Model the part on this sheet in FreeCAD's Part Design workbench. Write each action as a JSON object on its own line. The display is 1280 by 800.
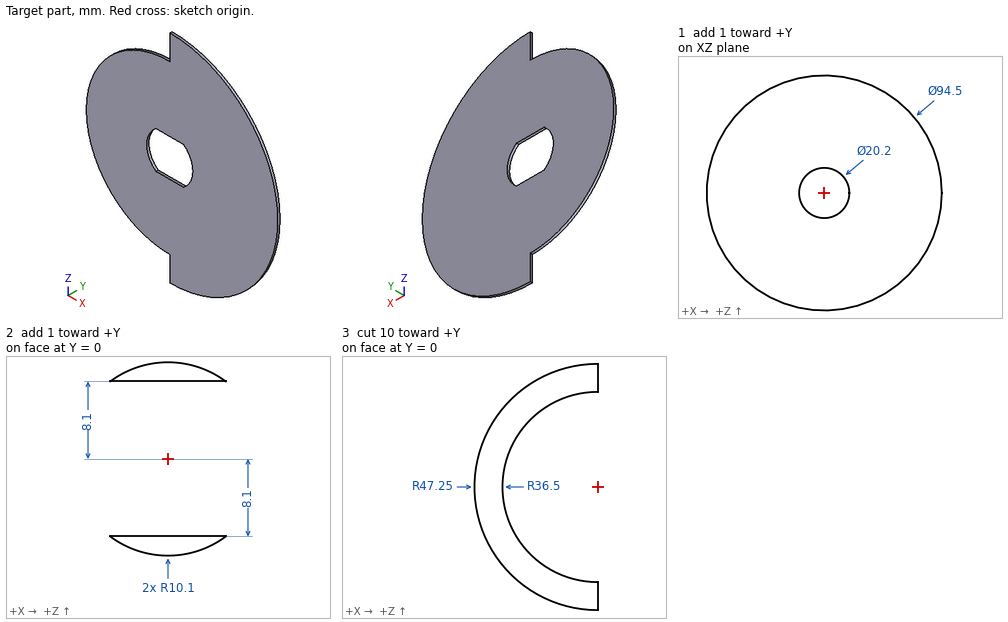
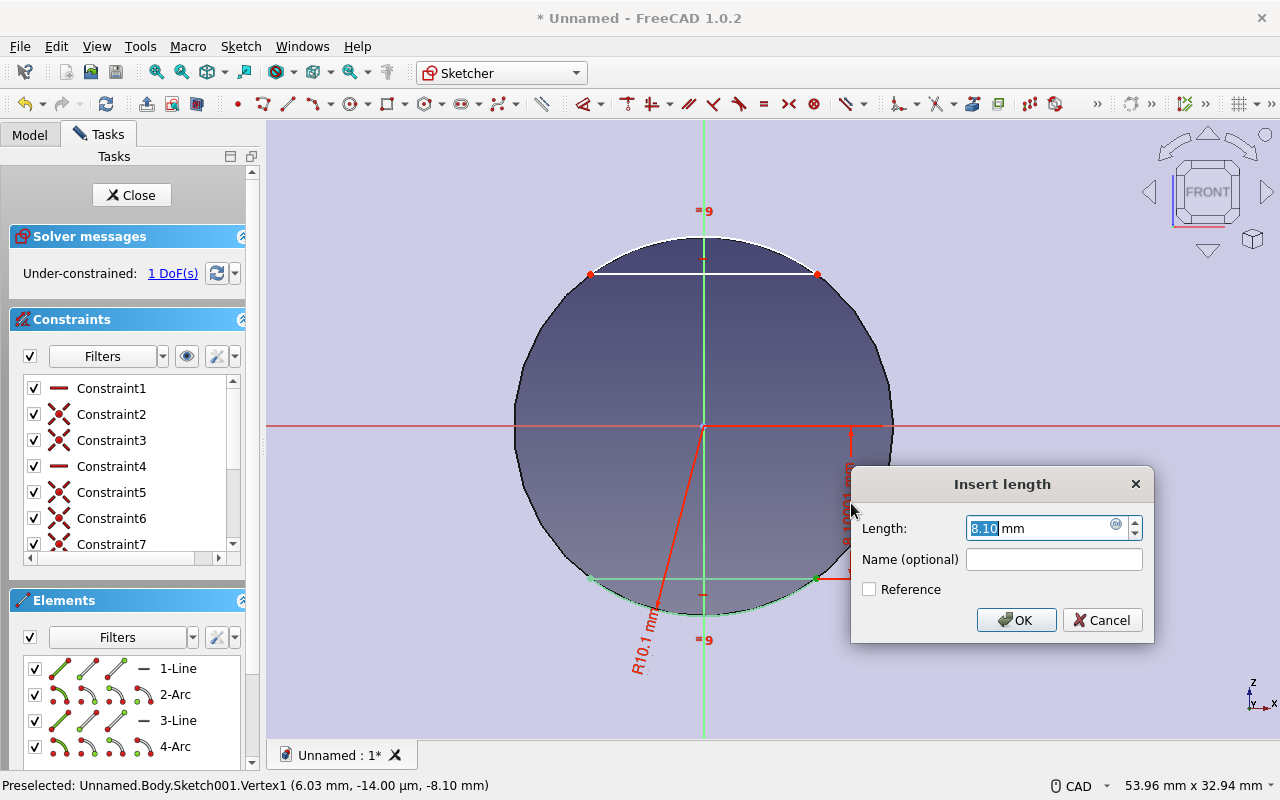
{"action": "type", "text": "8.1"}
{"action": "key", "text": "Return"}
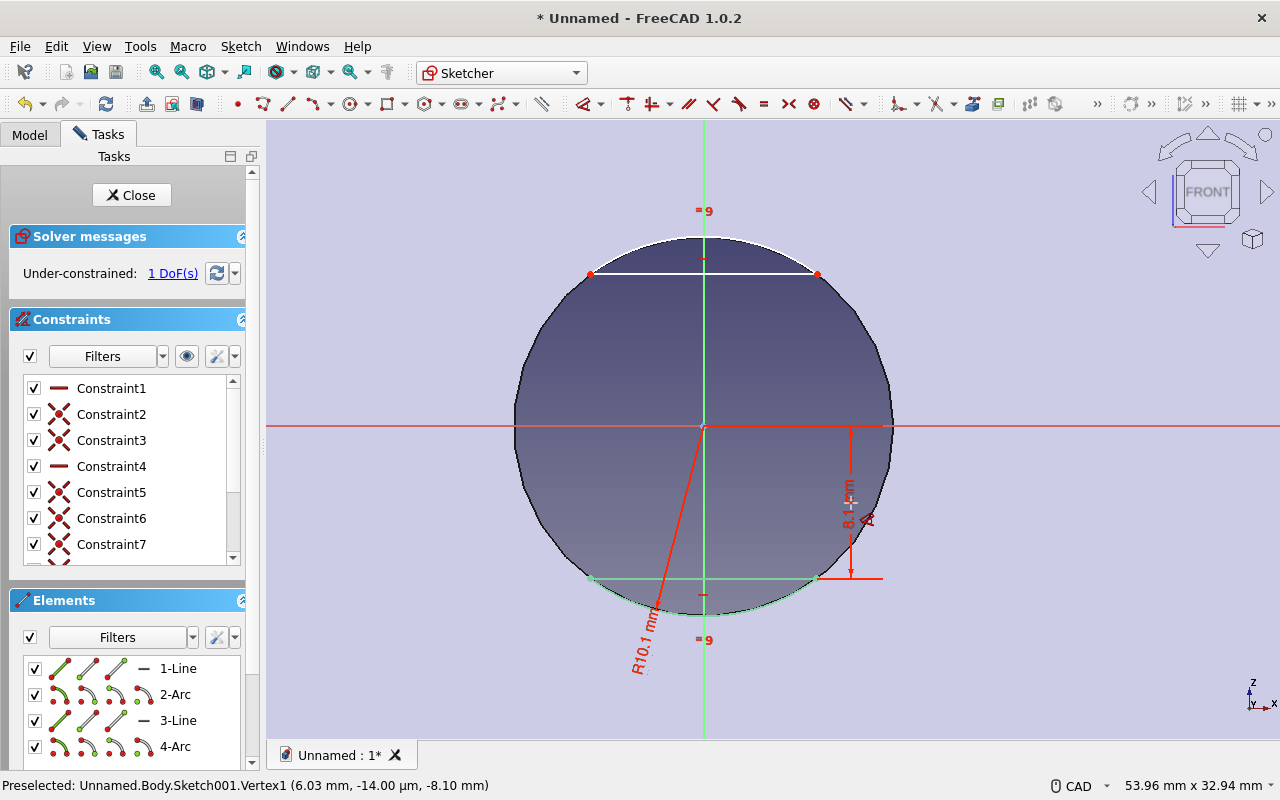
{"action": "left_click", "coordinate": [590, 274]}
{"action": "left_click", "coordinate": [556, 350]}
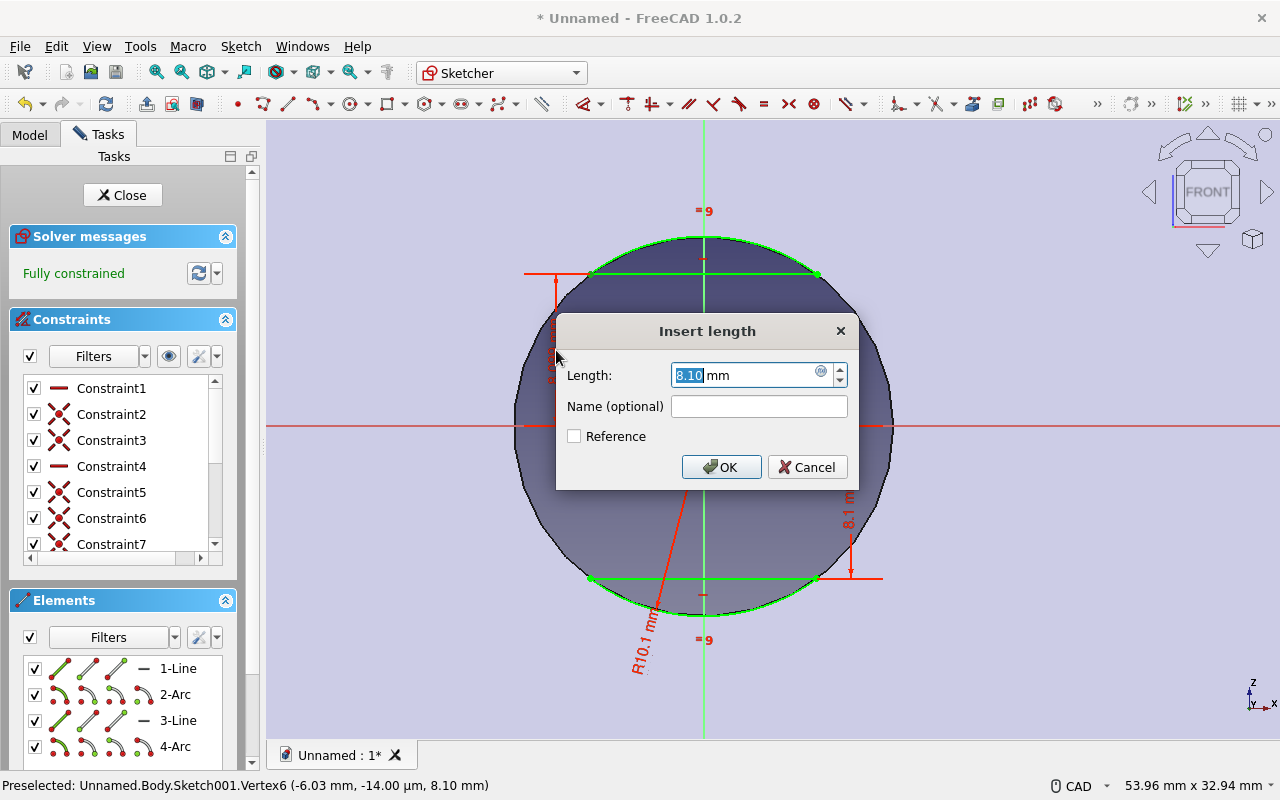
{"action": "type", "text": "8.1"}
{"action": "key", "text": "Return"}
{"action": "key", "text": "Escape"}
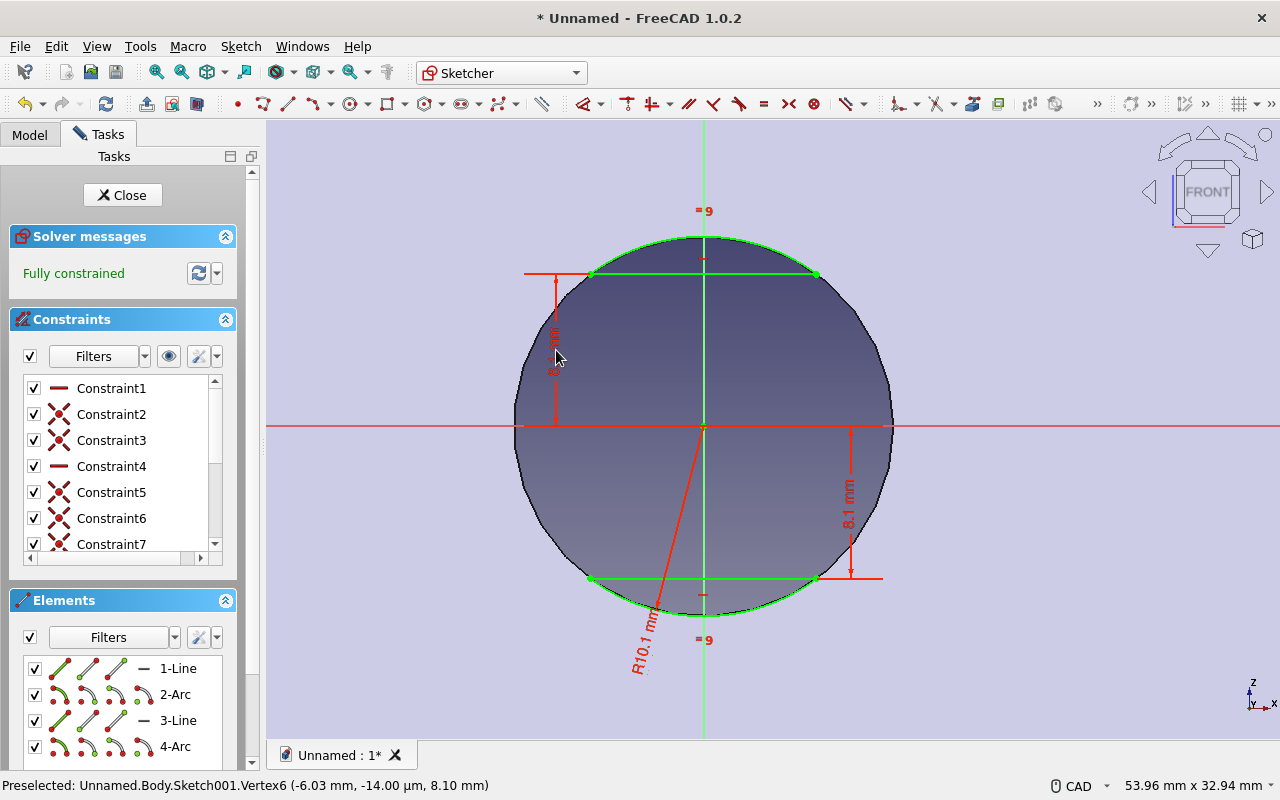
{"action": "left_click", "coordinate": [123, 195]}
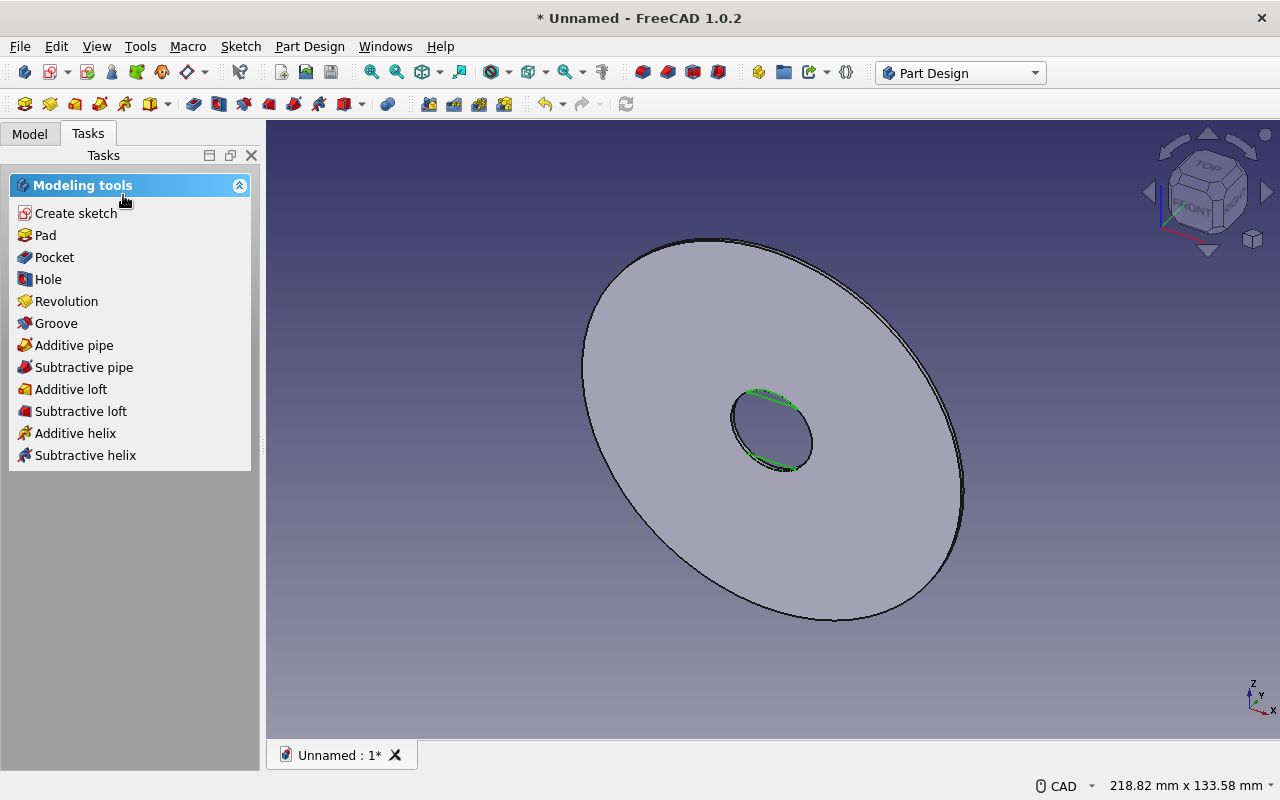
{"action": "left_click", "coordinate": [25, 104]}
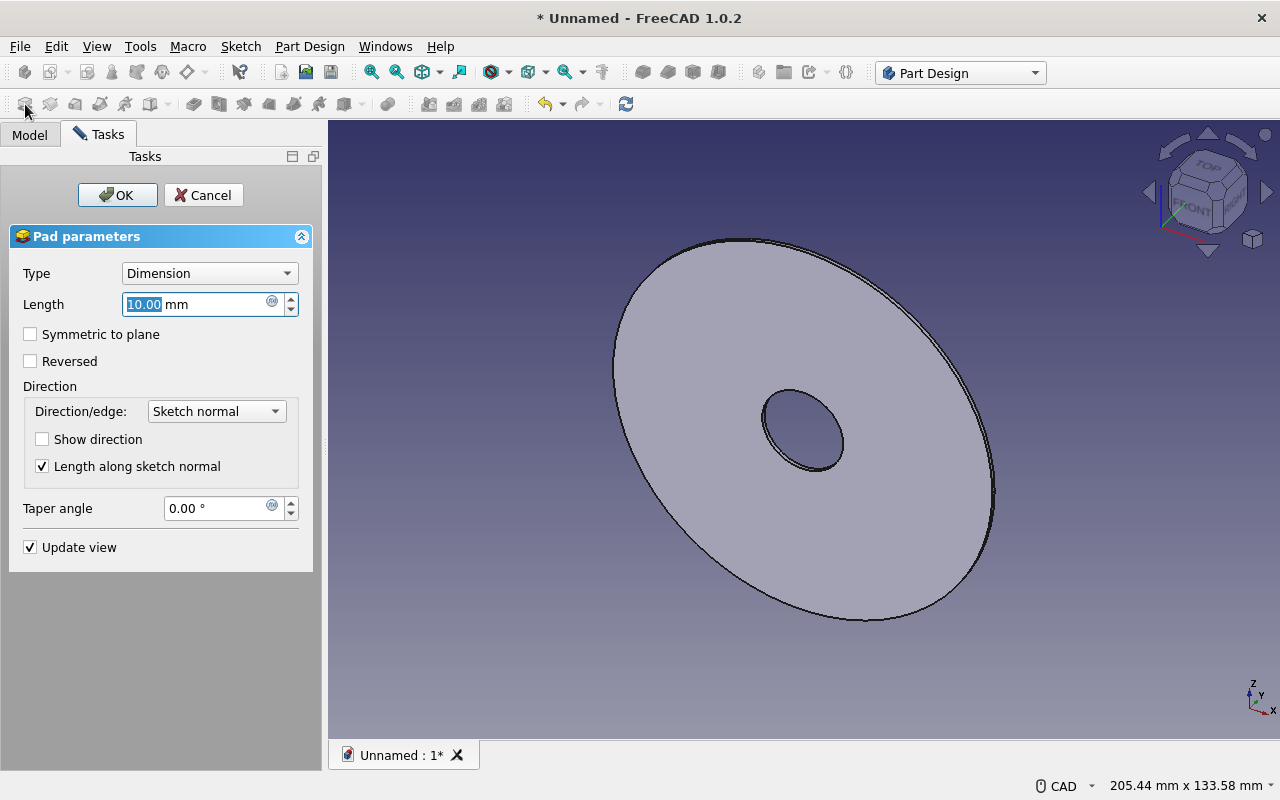
{"action": "type", "text": "1"}
{"action": "key", "text": "Tab"}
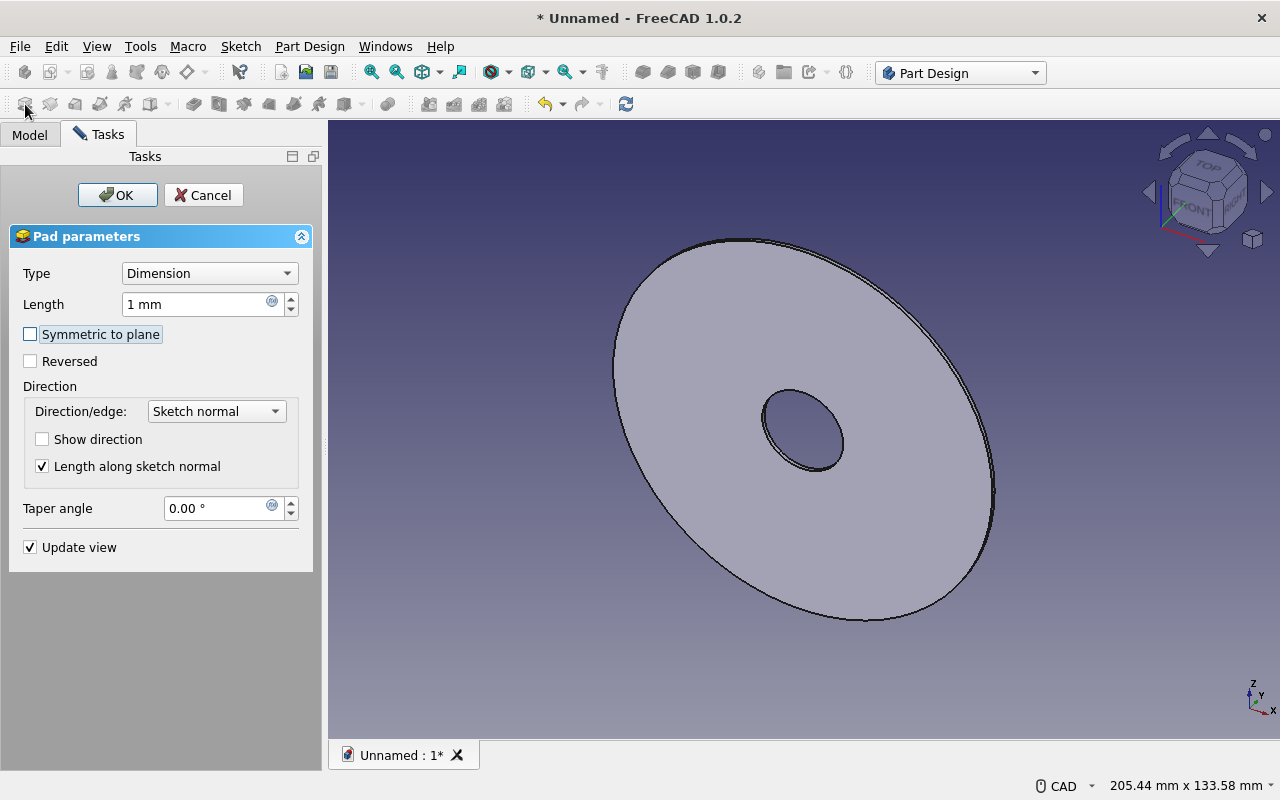
{"action": "left_click", "coordinate": [31, 361]}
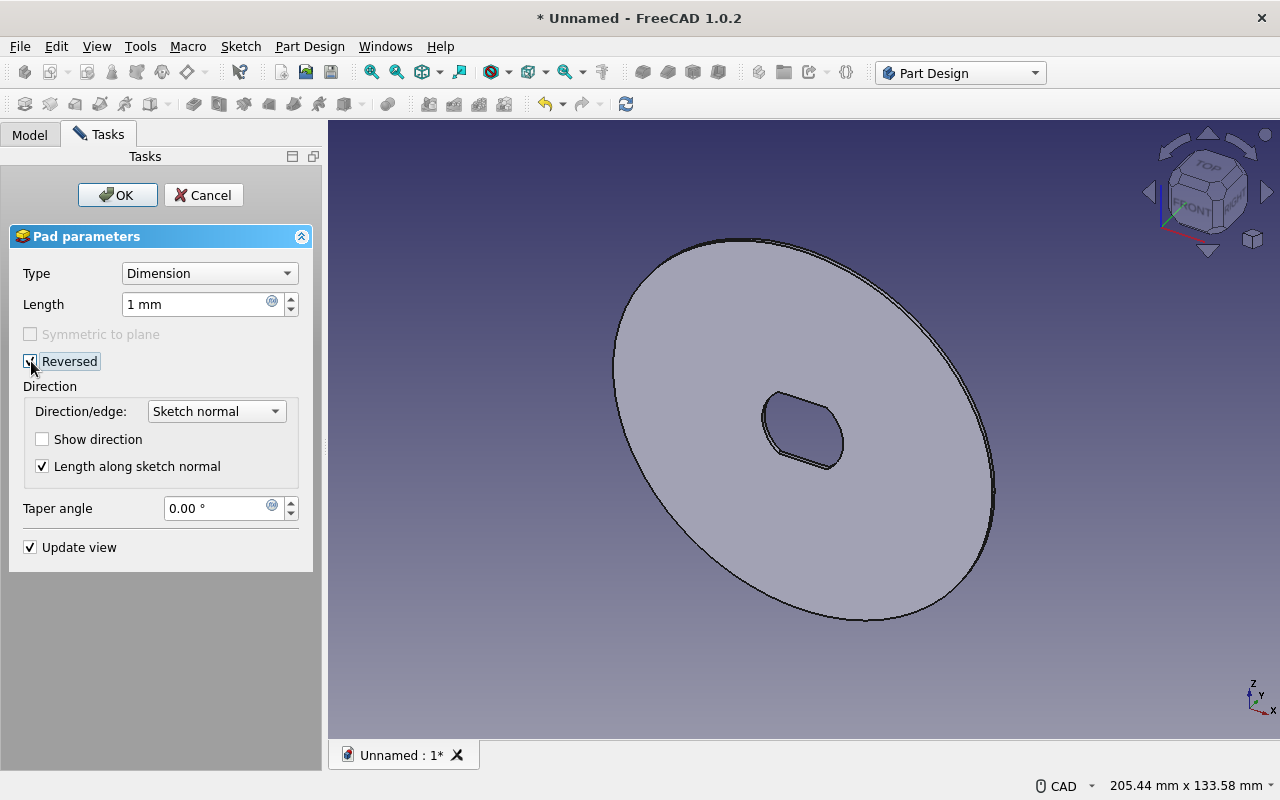
{"action": "left_click", "coordinate": [118, 195]}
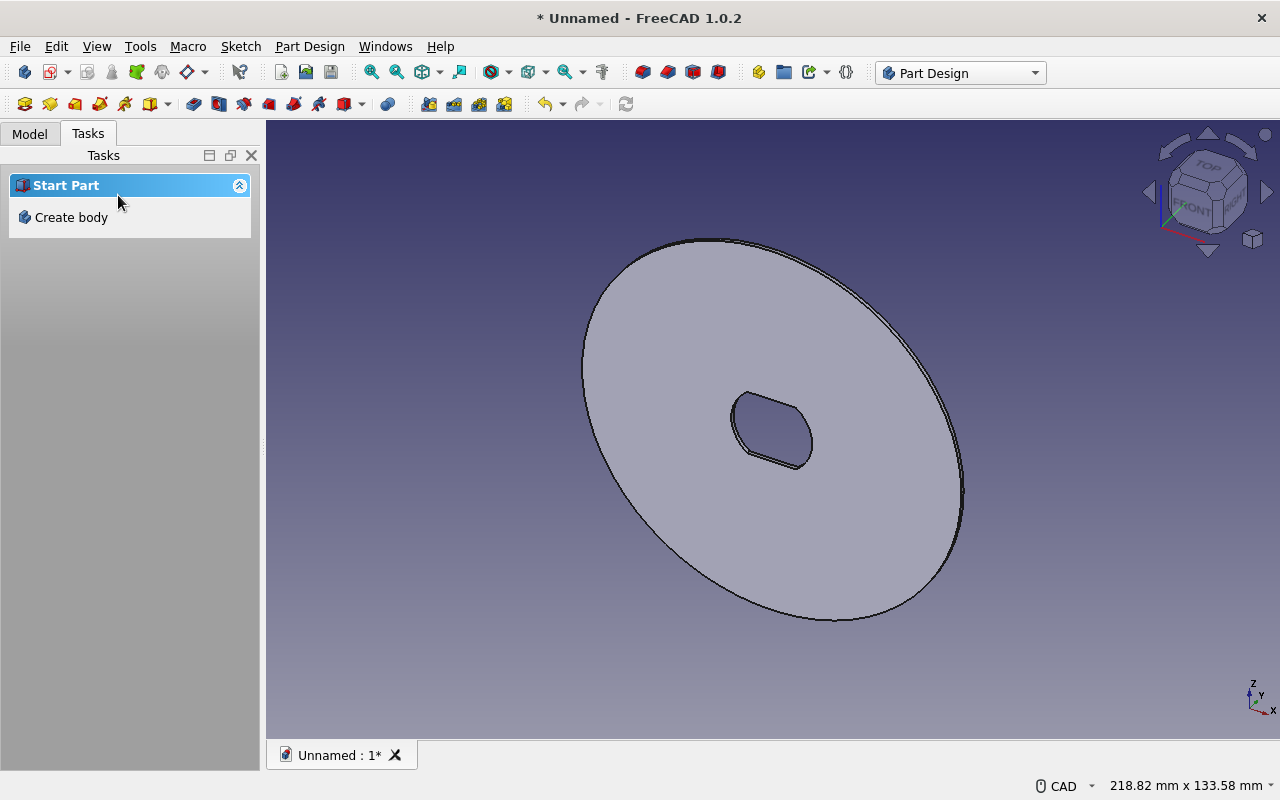
{"action": "left_click", "coordinate": [772, 532]}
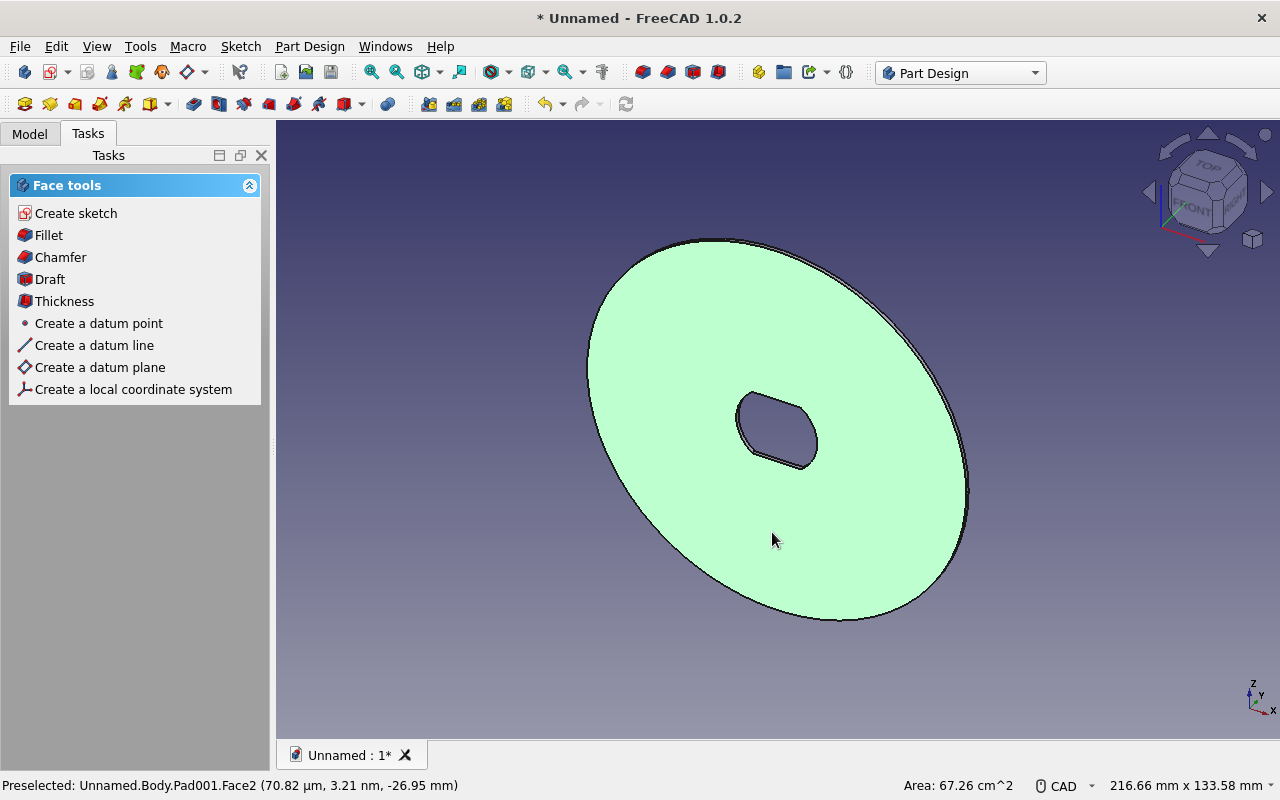
{"action": "left_click", "coordinate": [50, 72]}